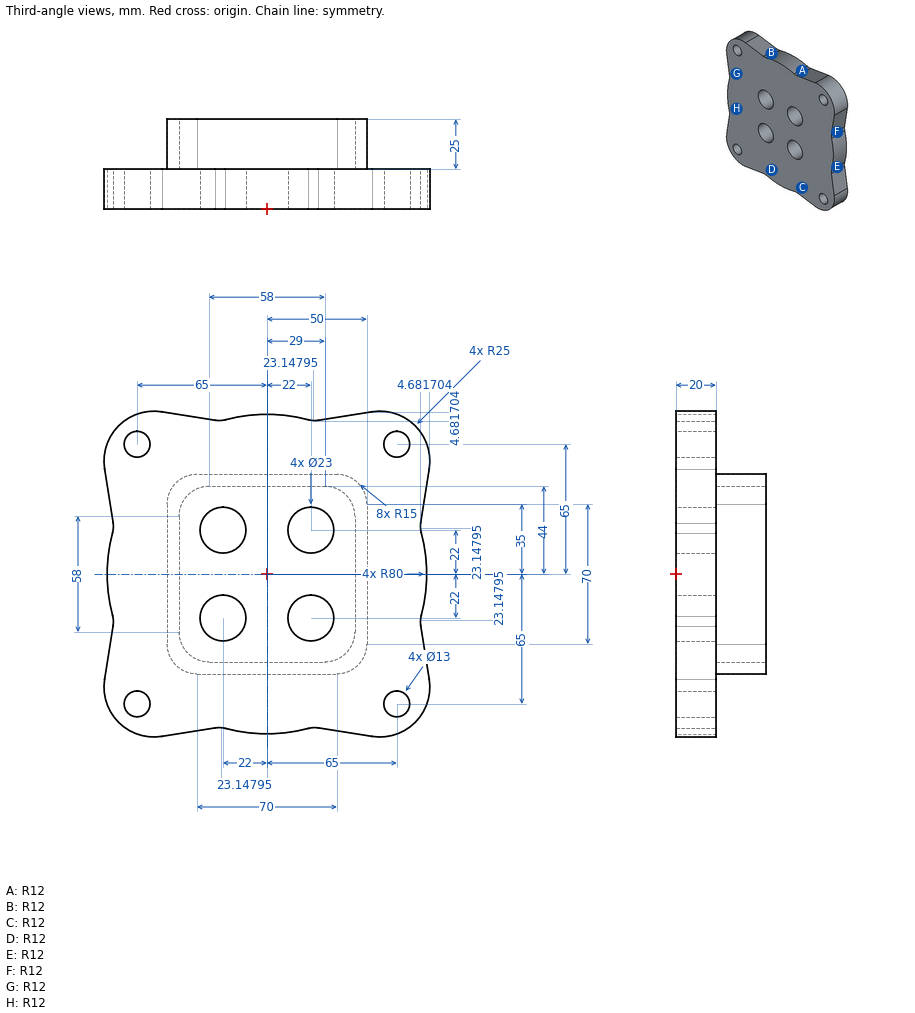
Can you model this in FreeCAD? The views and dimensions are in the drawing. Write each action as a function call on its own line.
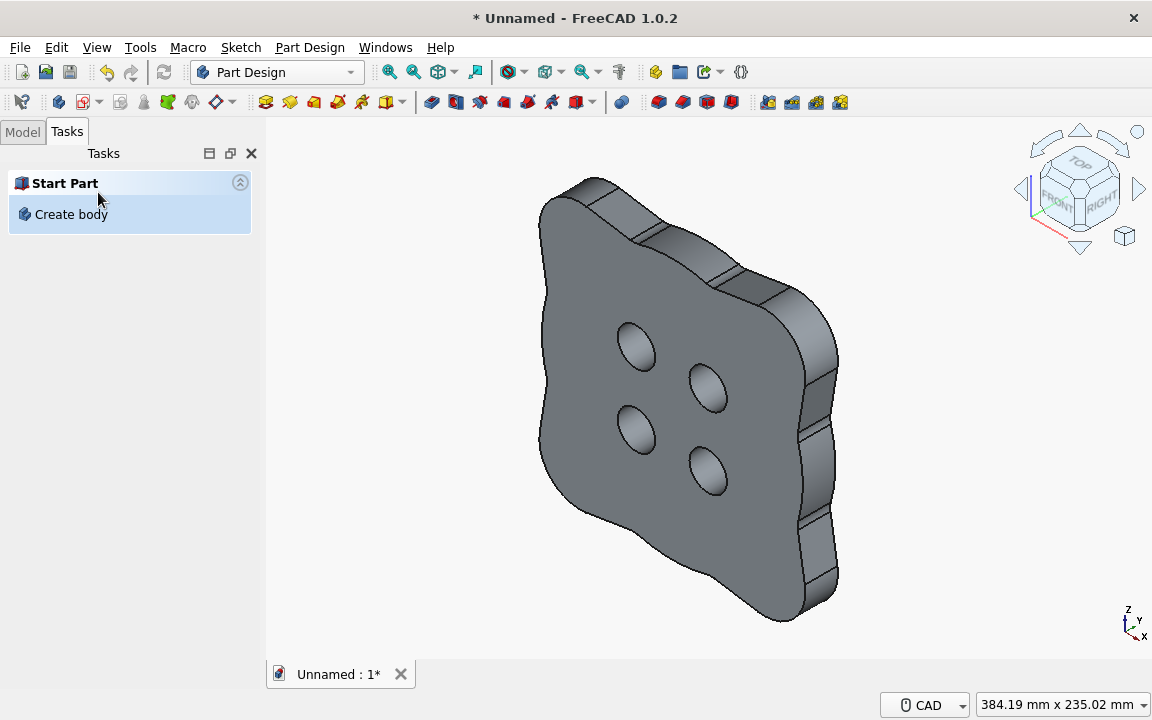
key(2)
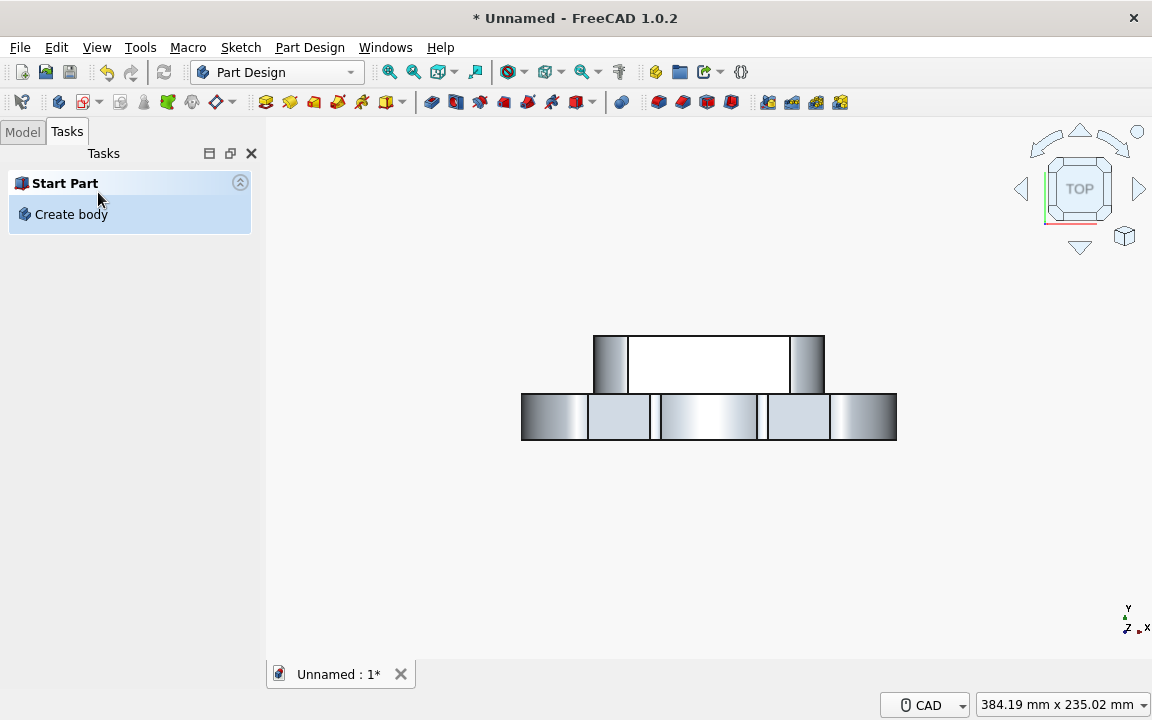
click(390, 72)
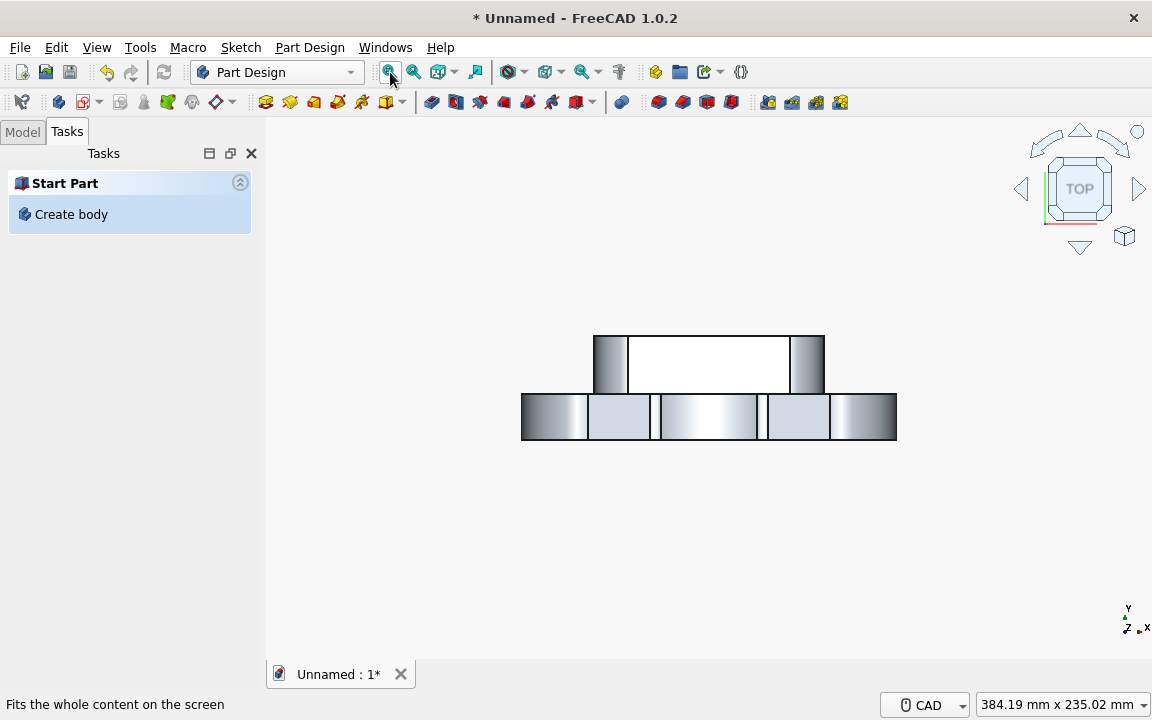
key(0)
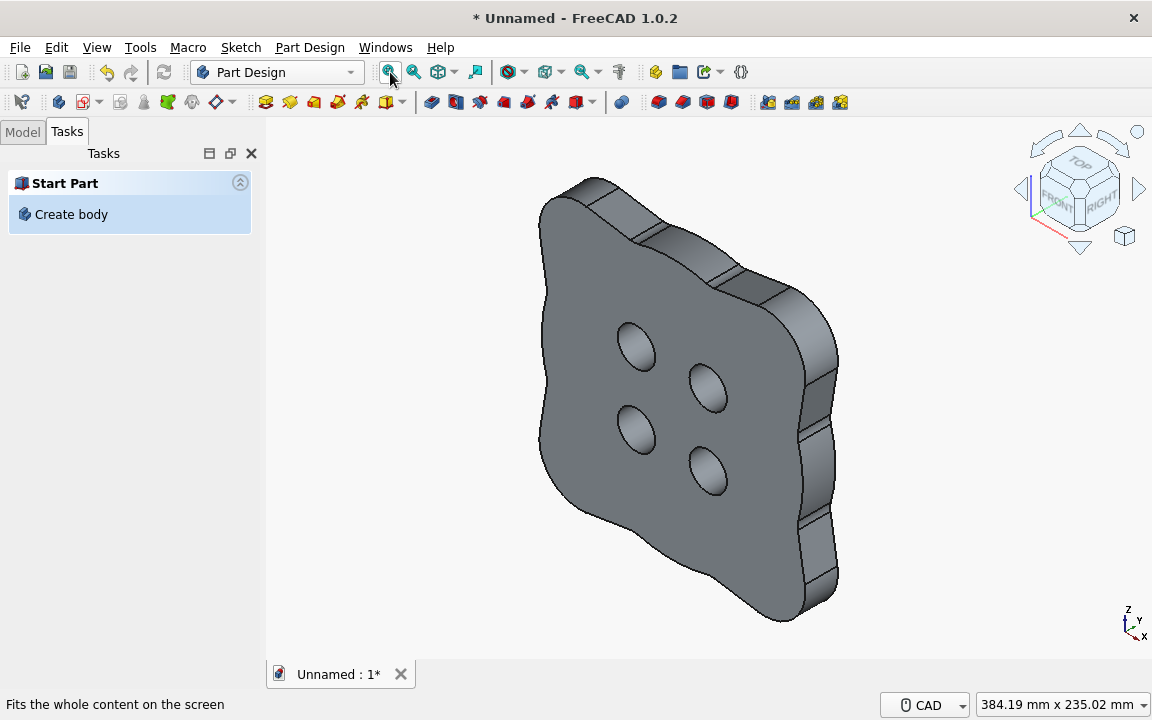
key(1)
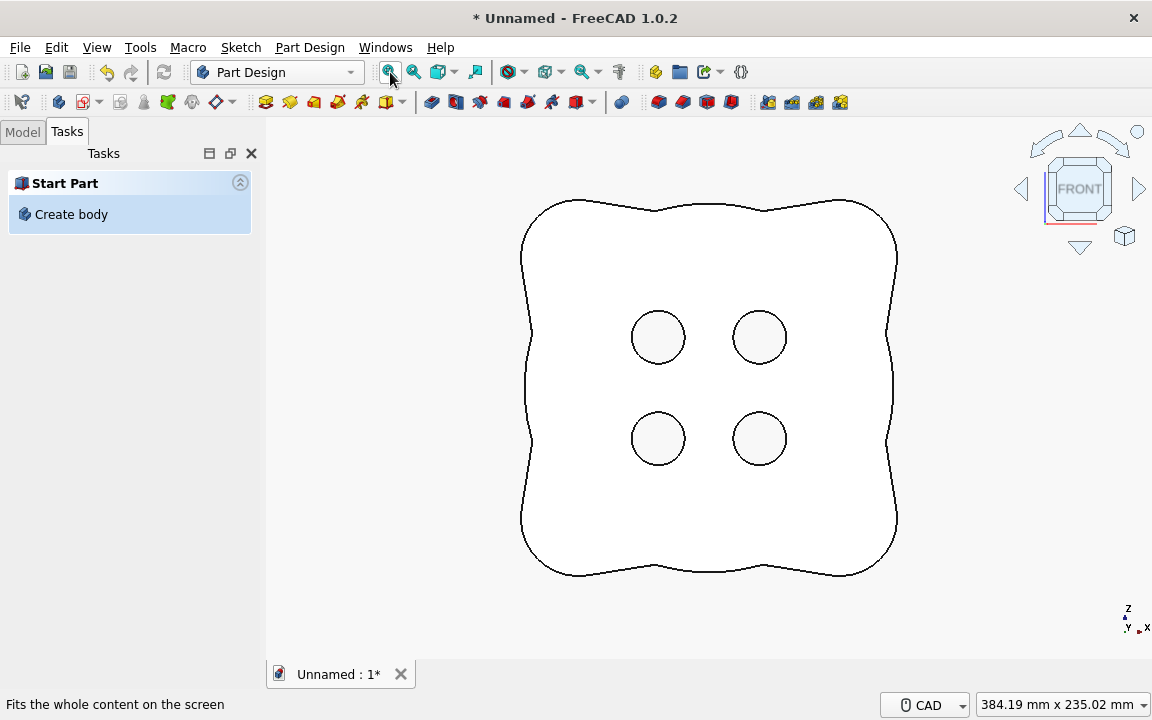
key(3)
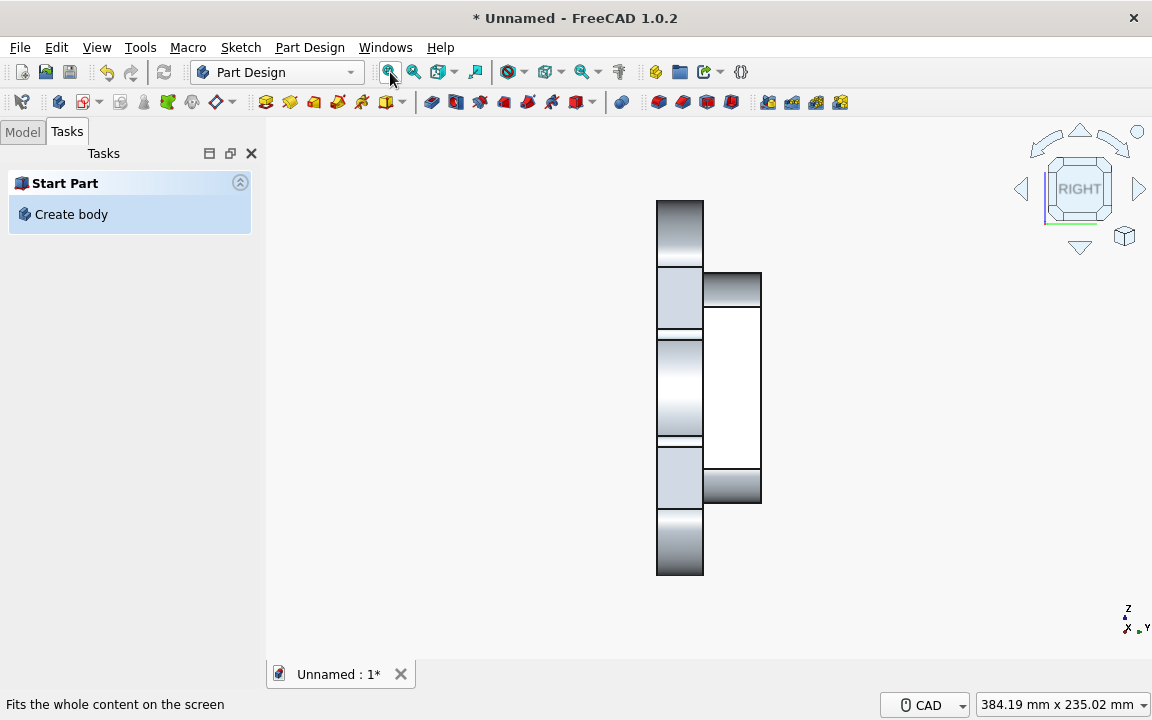
key(5)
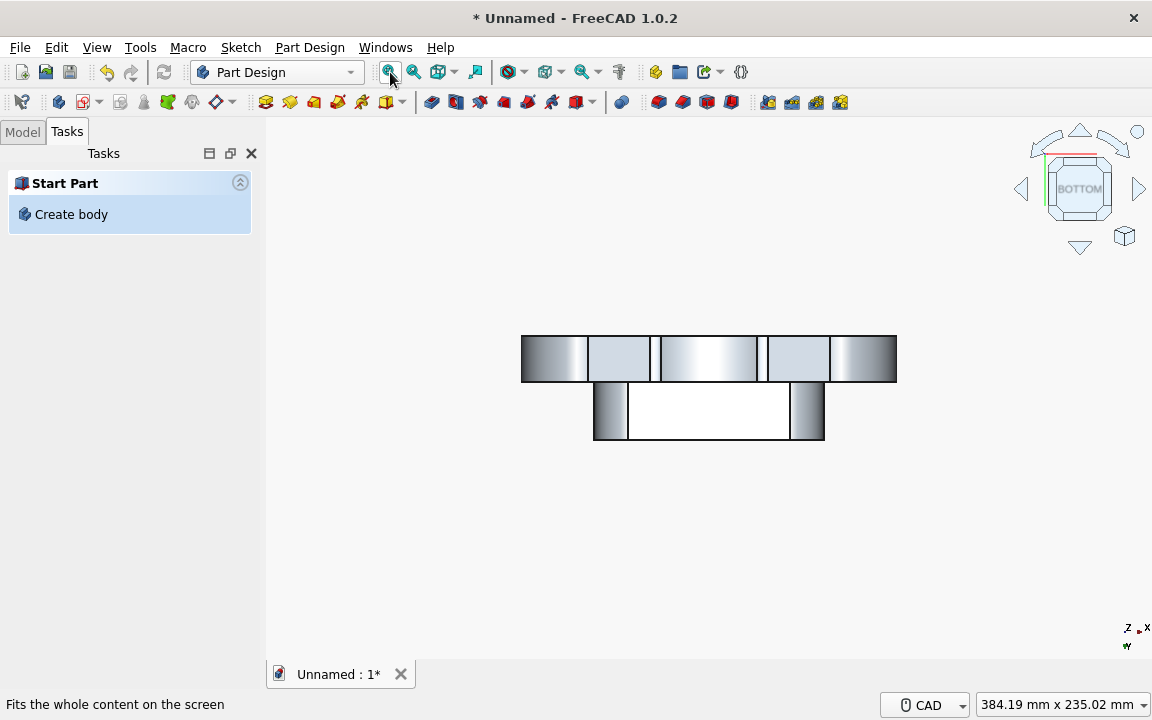
click(390, 72)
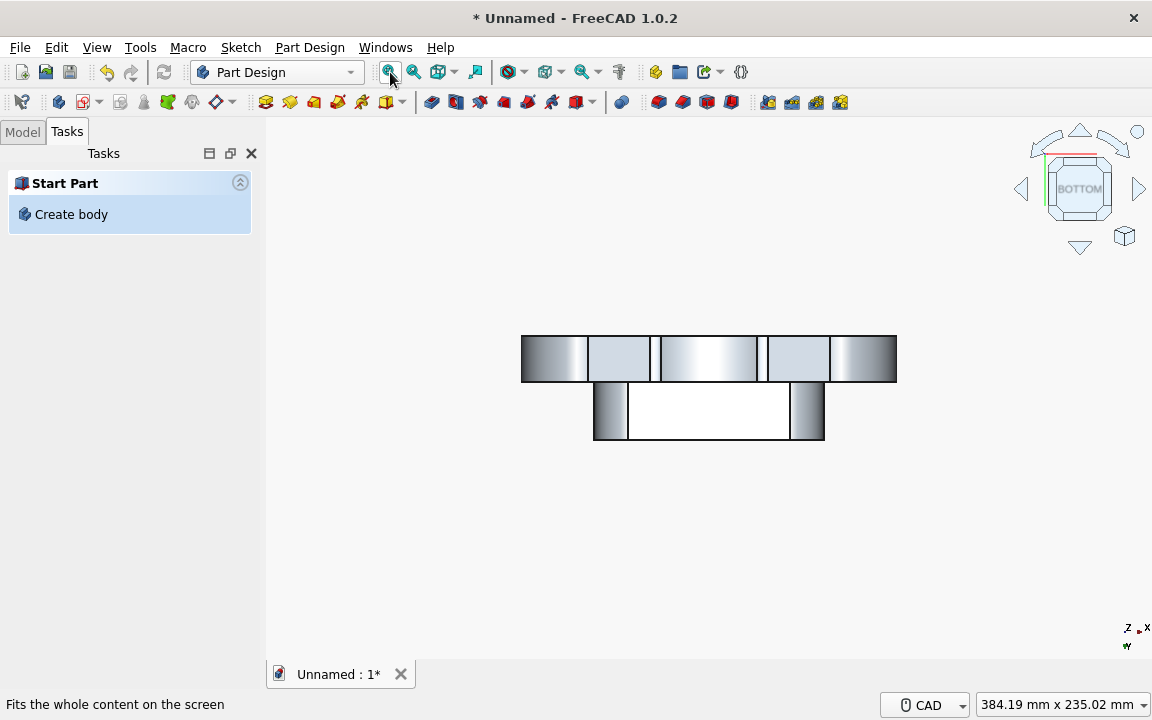
key(4)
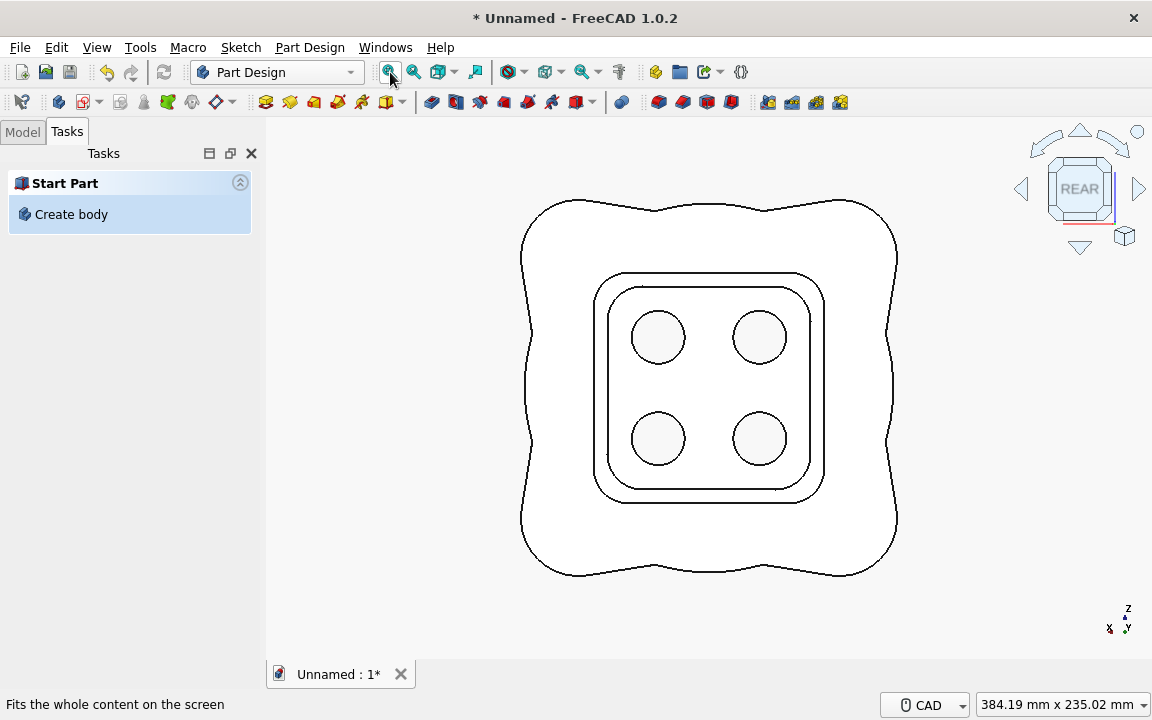
key(6)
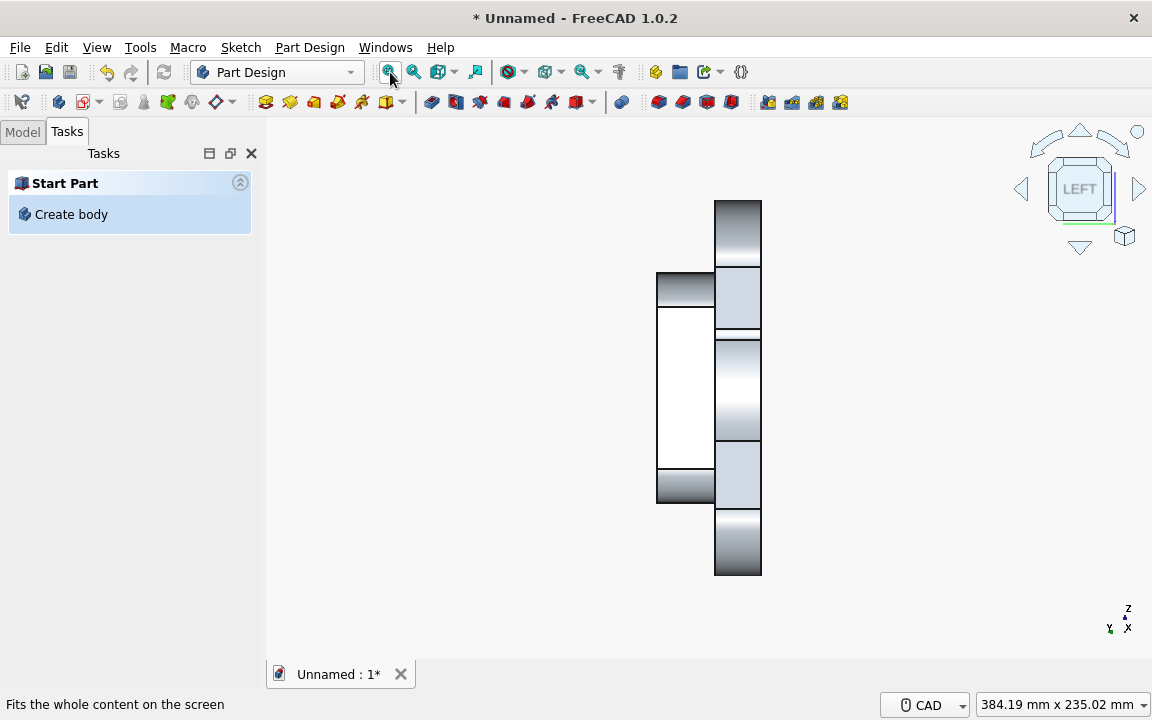
key(v)
key(3)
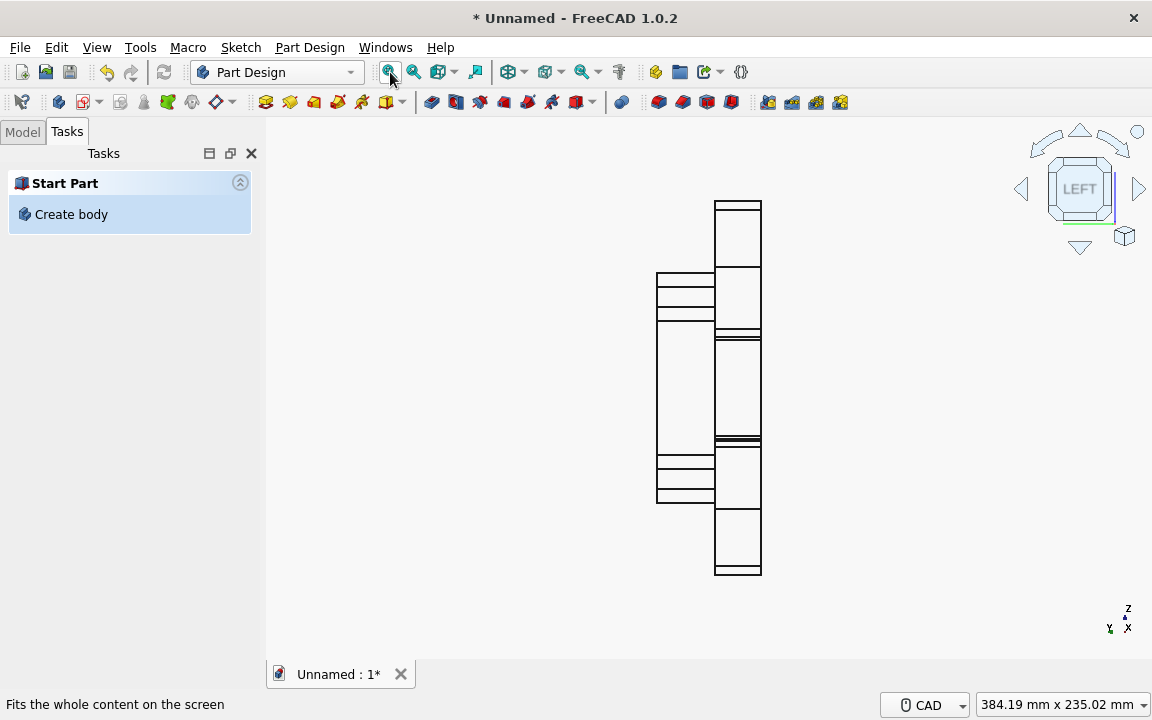
key(0)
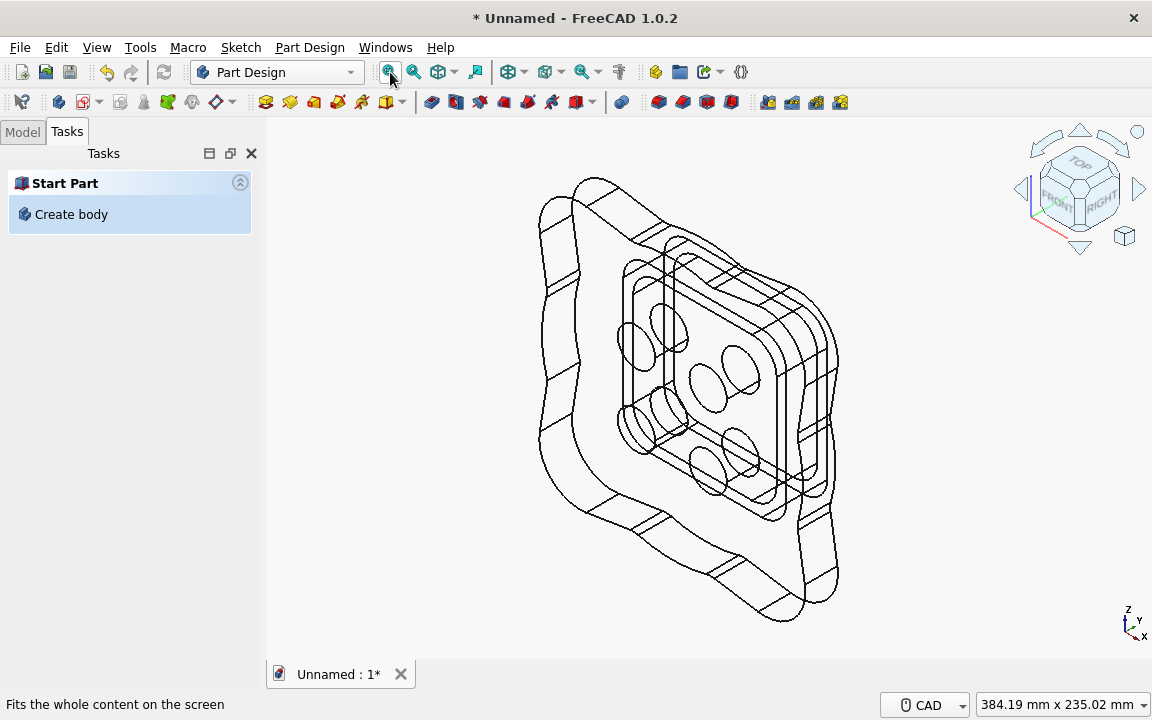
click(564, 370)